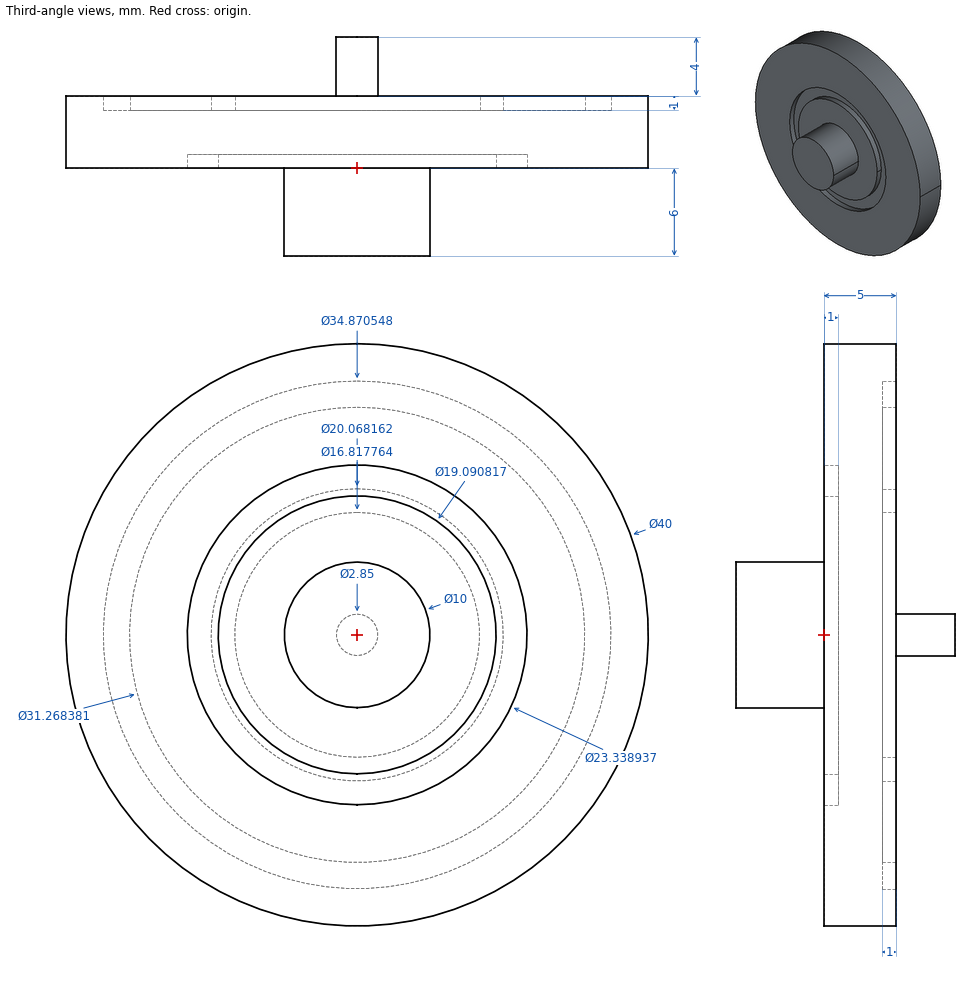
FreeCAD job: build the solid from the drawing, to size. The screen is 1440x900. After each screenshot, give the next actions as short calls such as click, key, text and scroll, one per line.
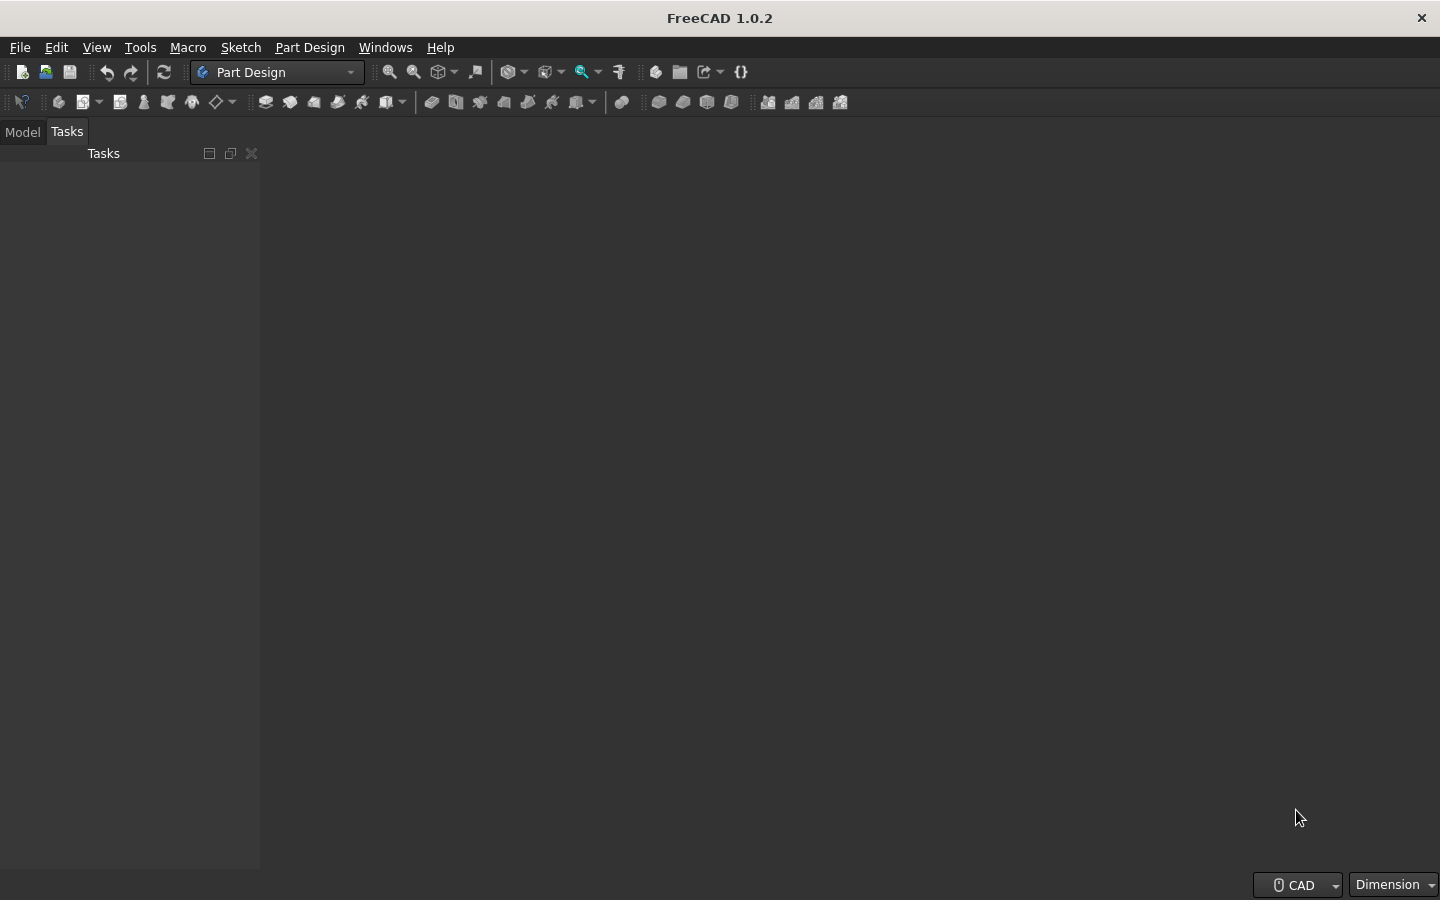
key(ctrl+n)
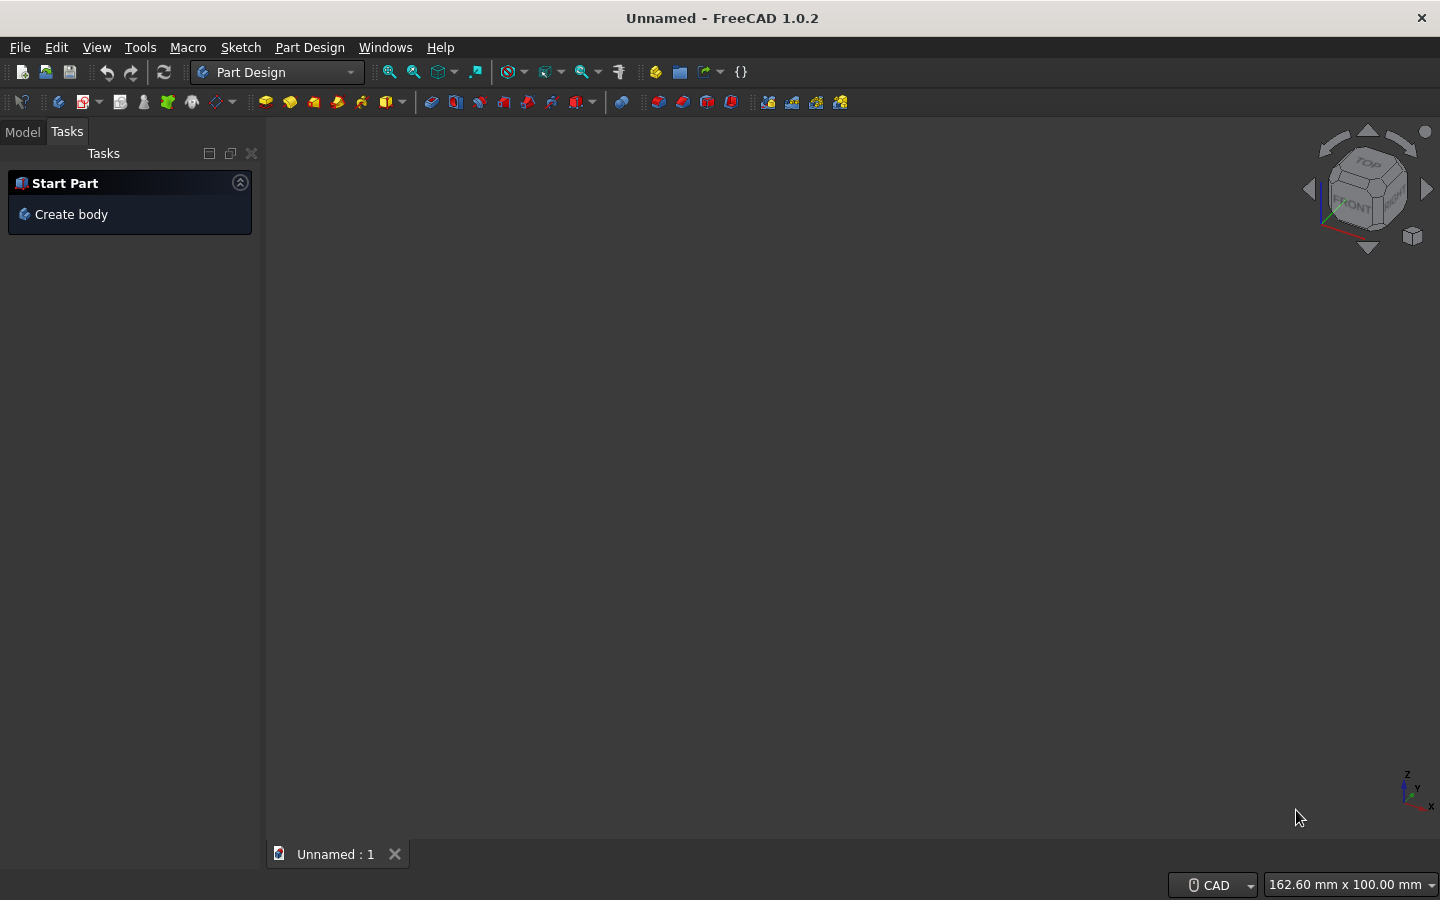
click(84, 102)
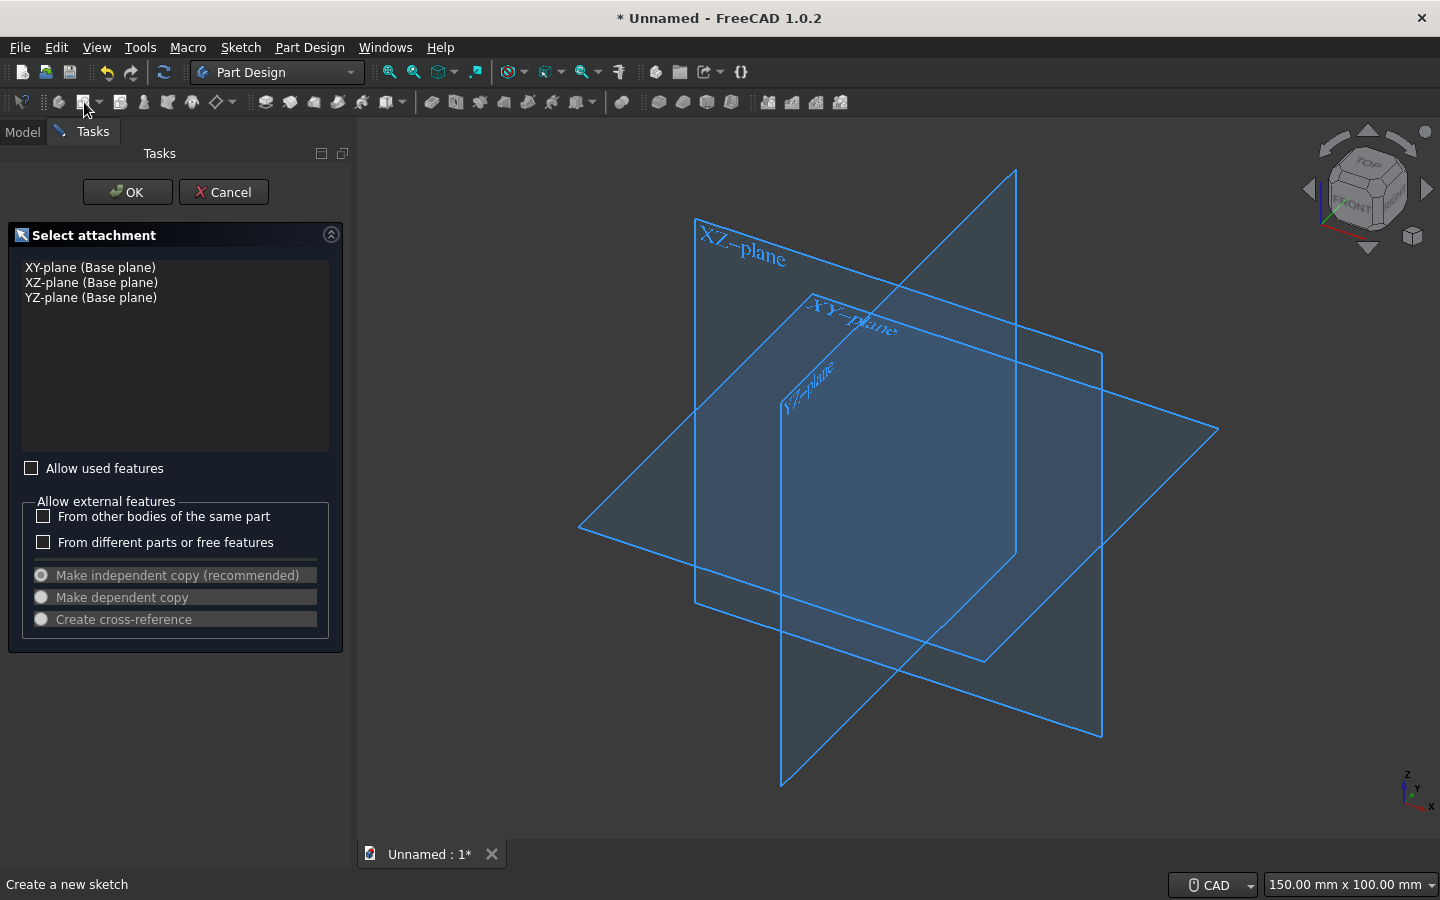
click(82, 282)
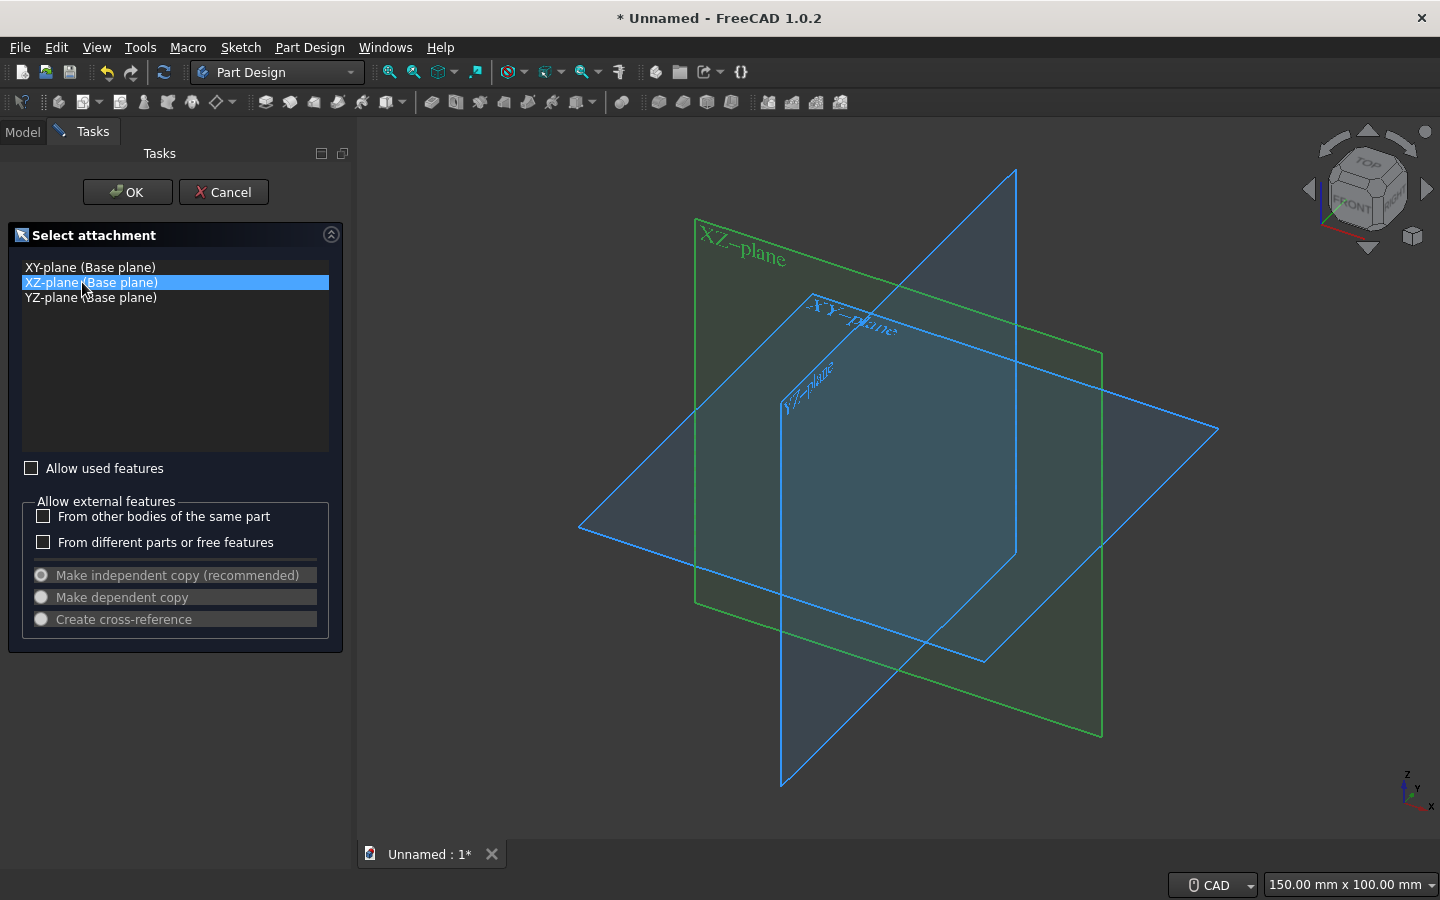
click(128, 192)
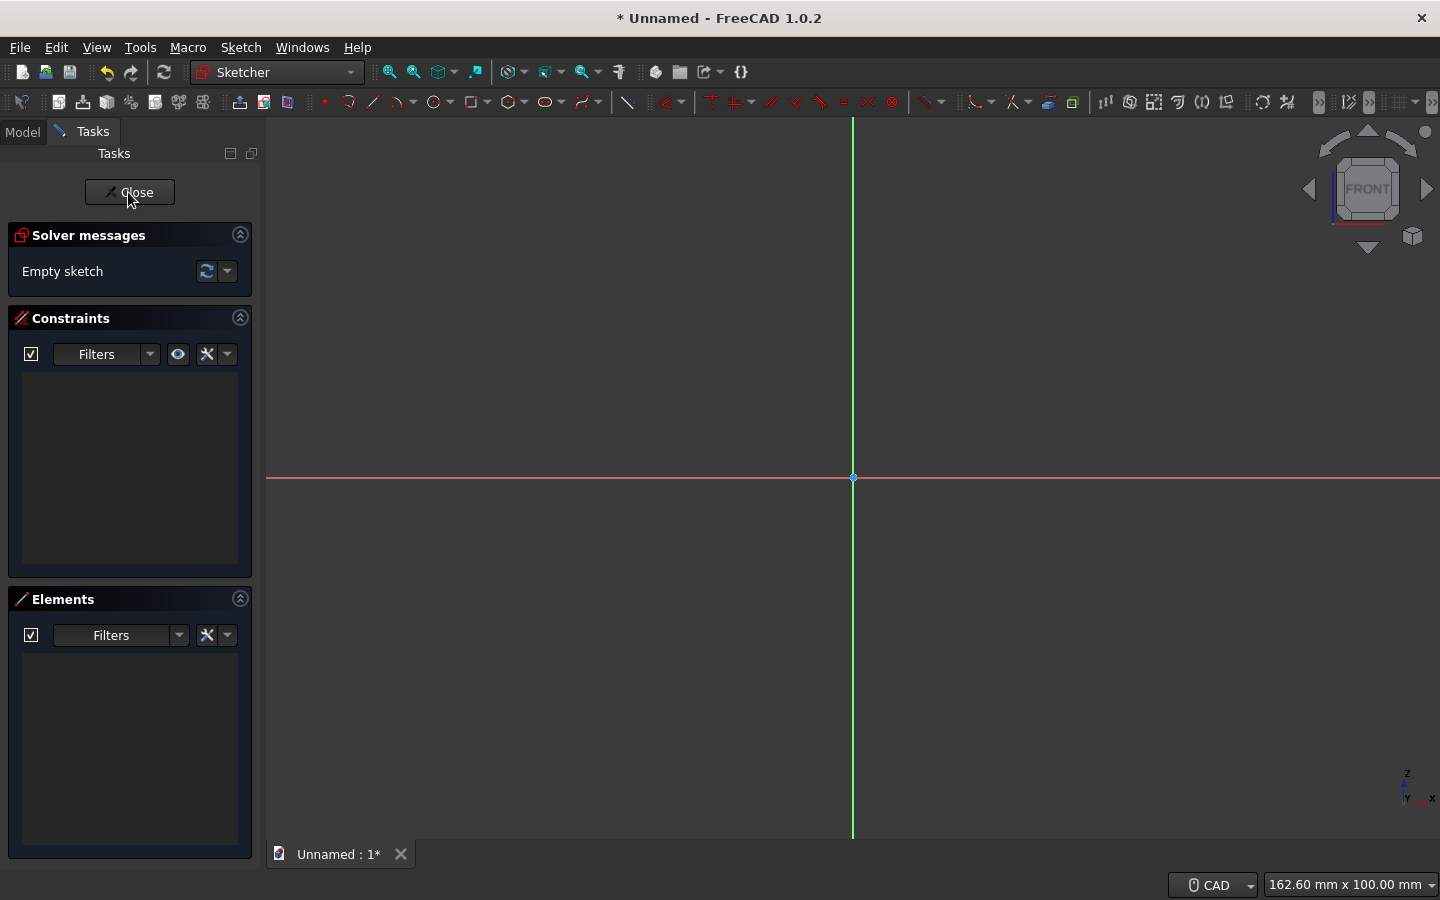
scroll(992, 478, up, 2)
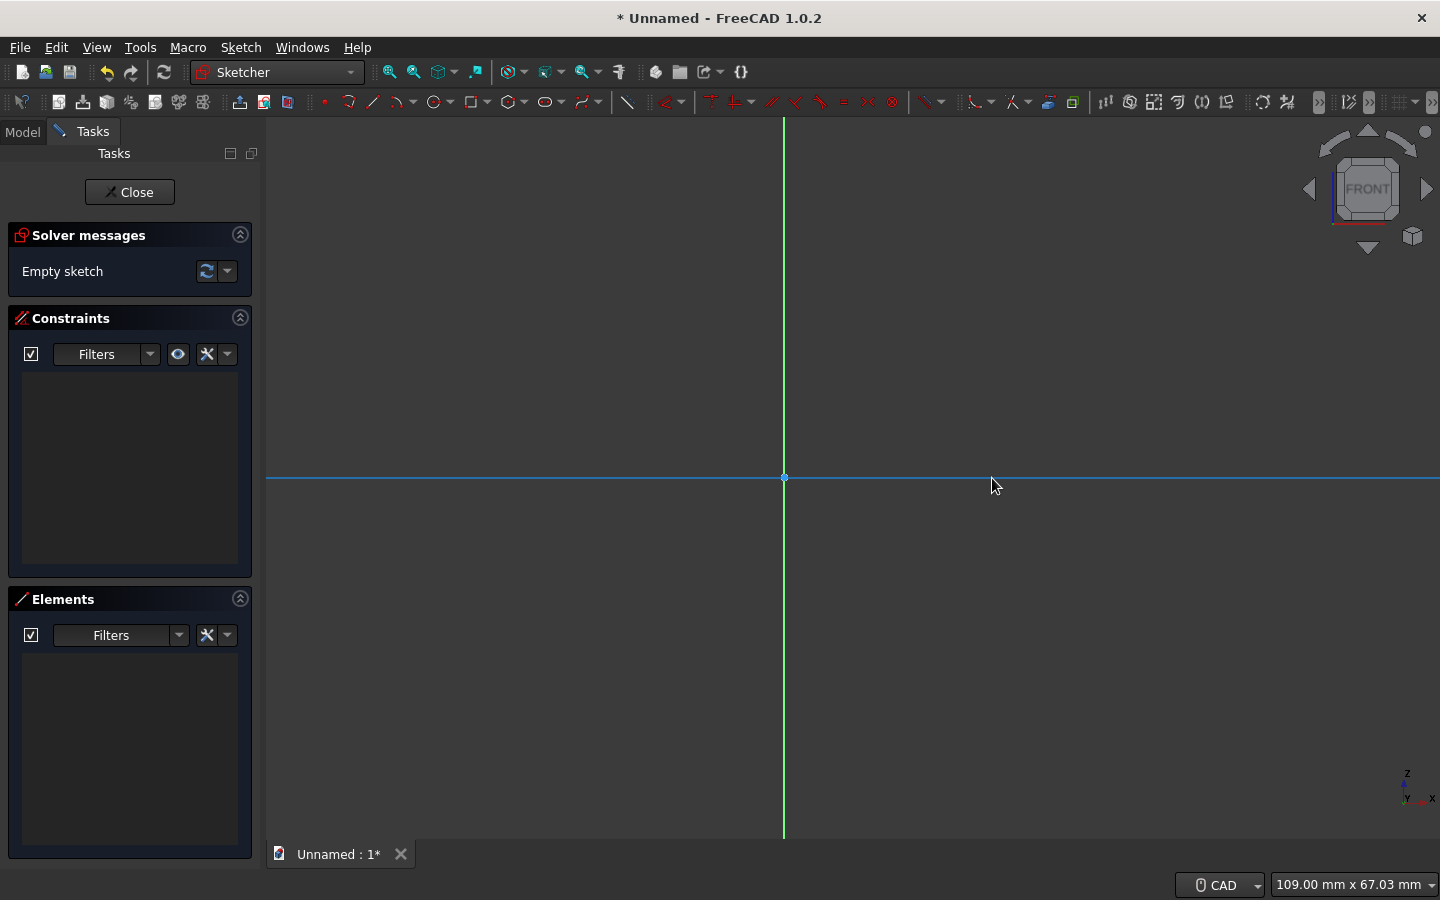
click(434, 102)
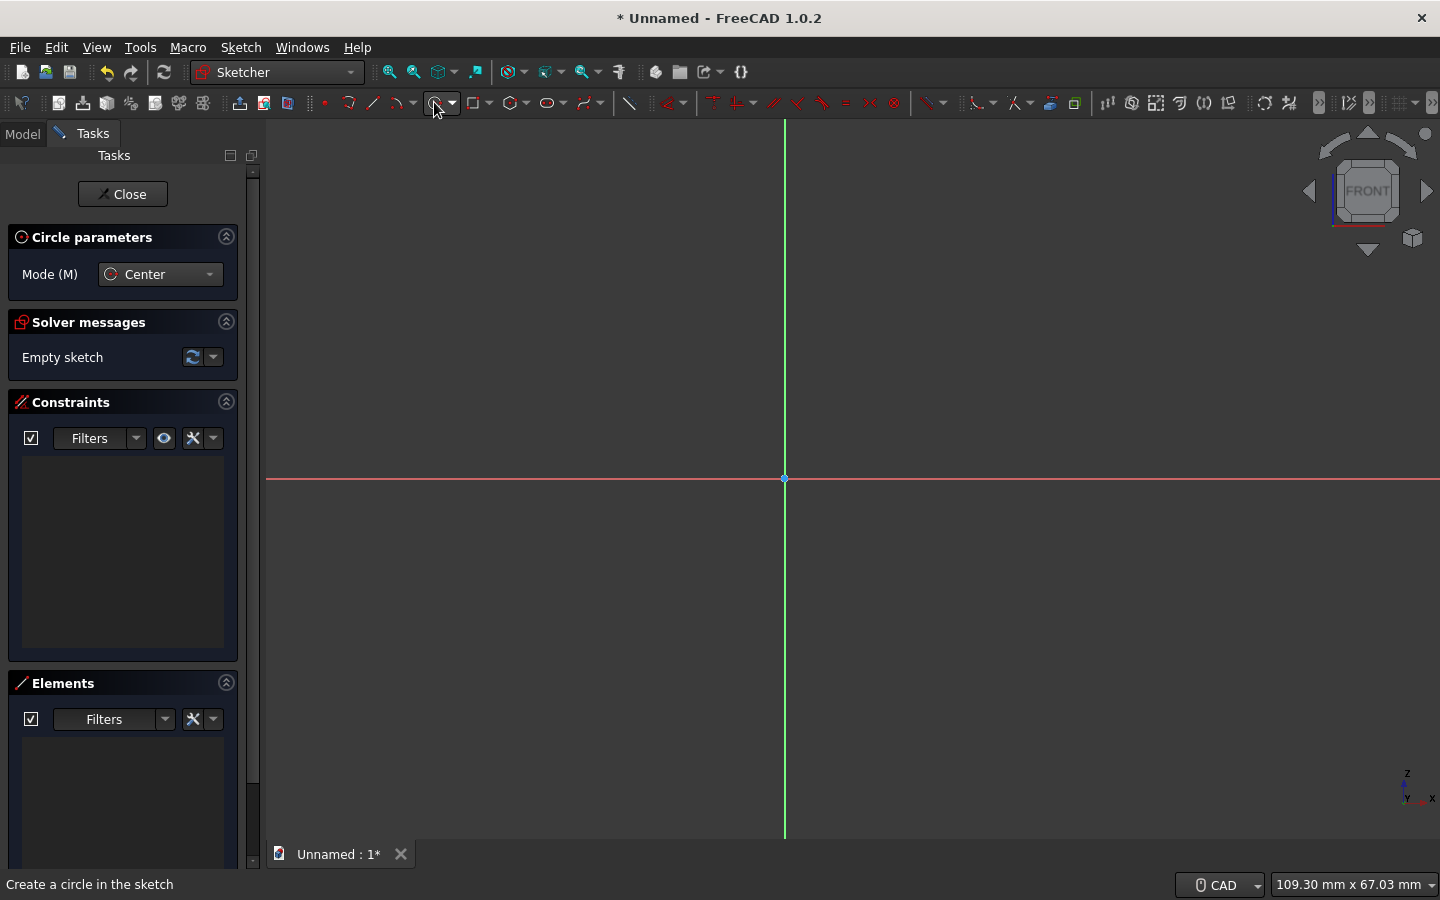
click(785, 479)
click(936, 327)
key(Escape)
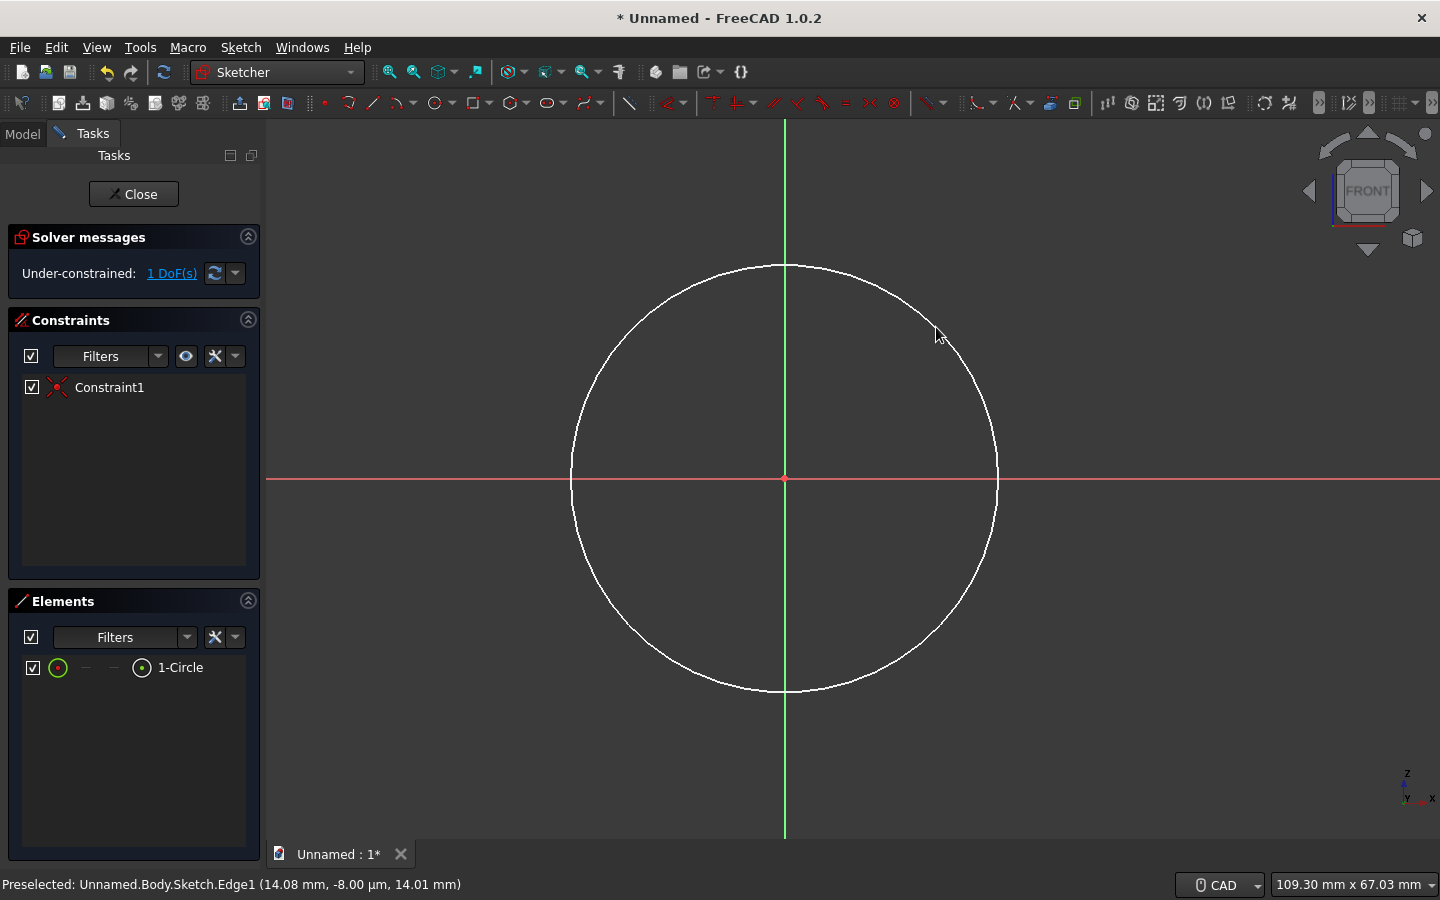
key(d)